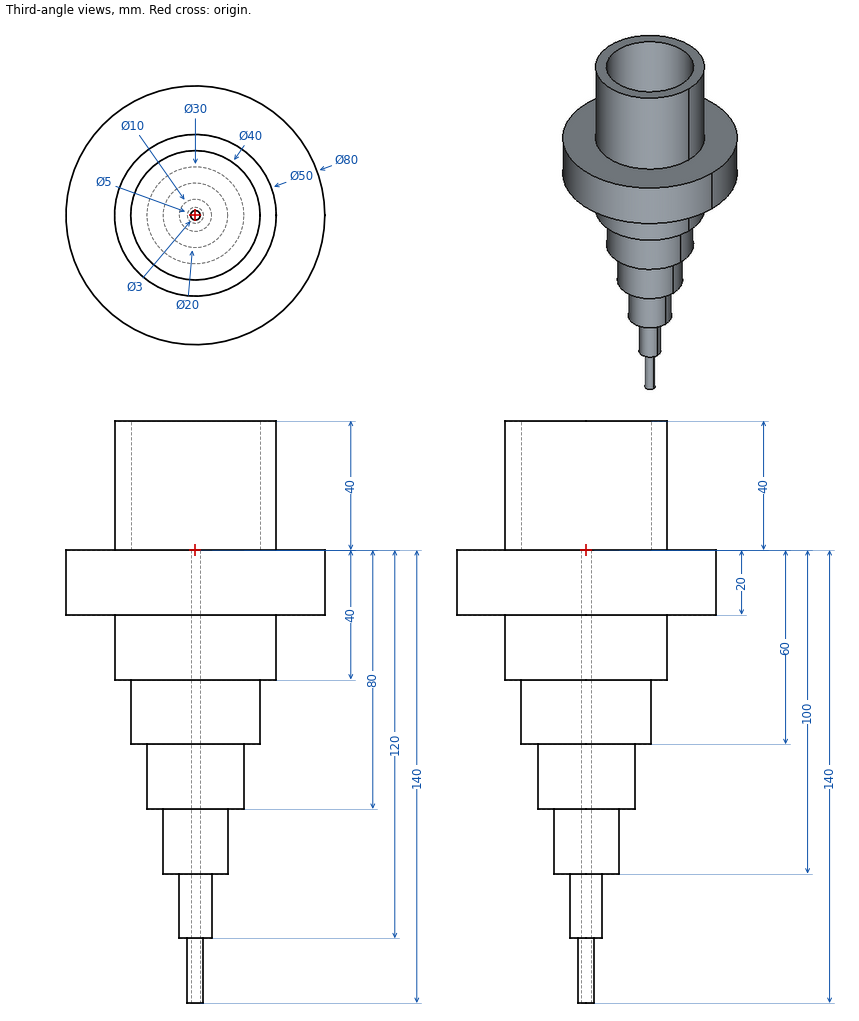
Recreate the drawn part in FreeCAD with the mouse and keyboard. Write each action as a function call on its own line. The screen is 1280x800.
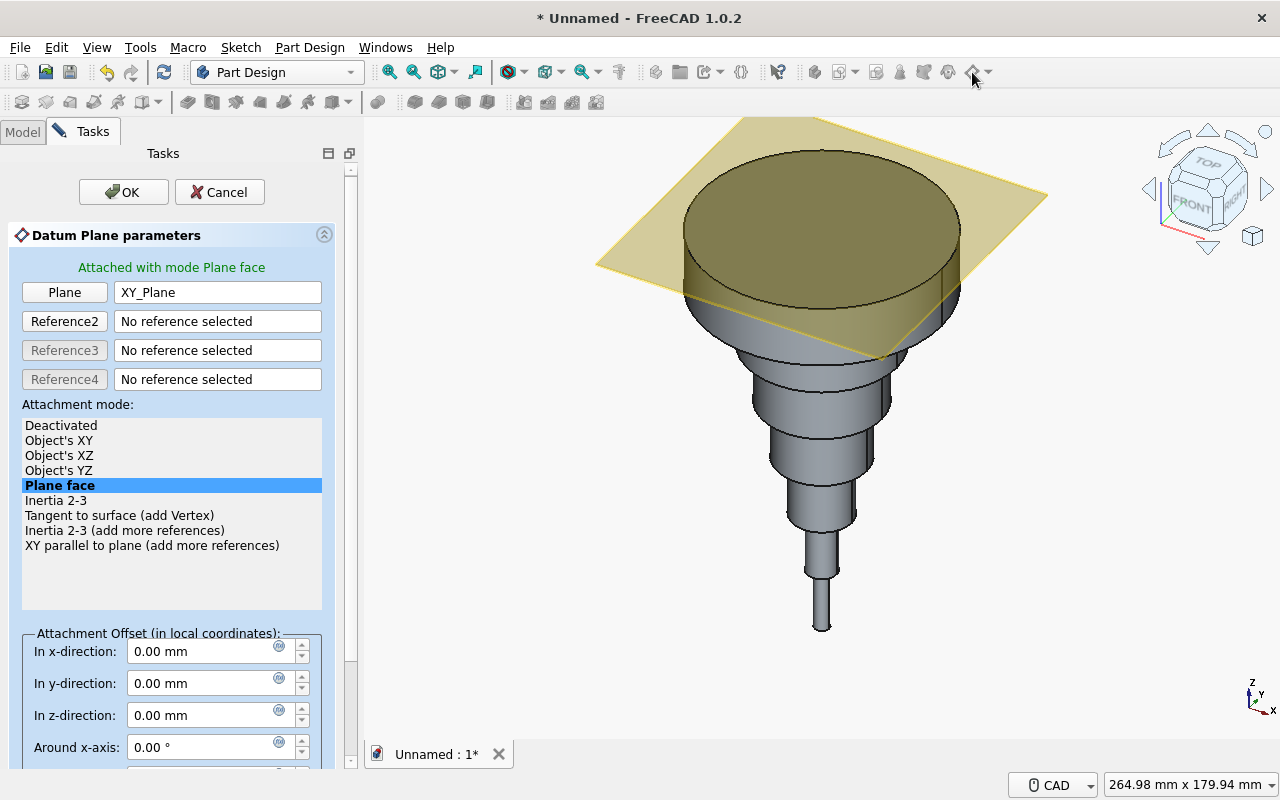
triple_click(210, 715)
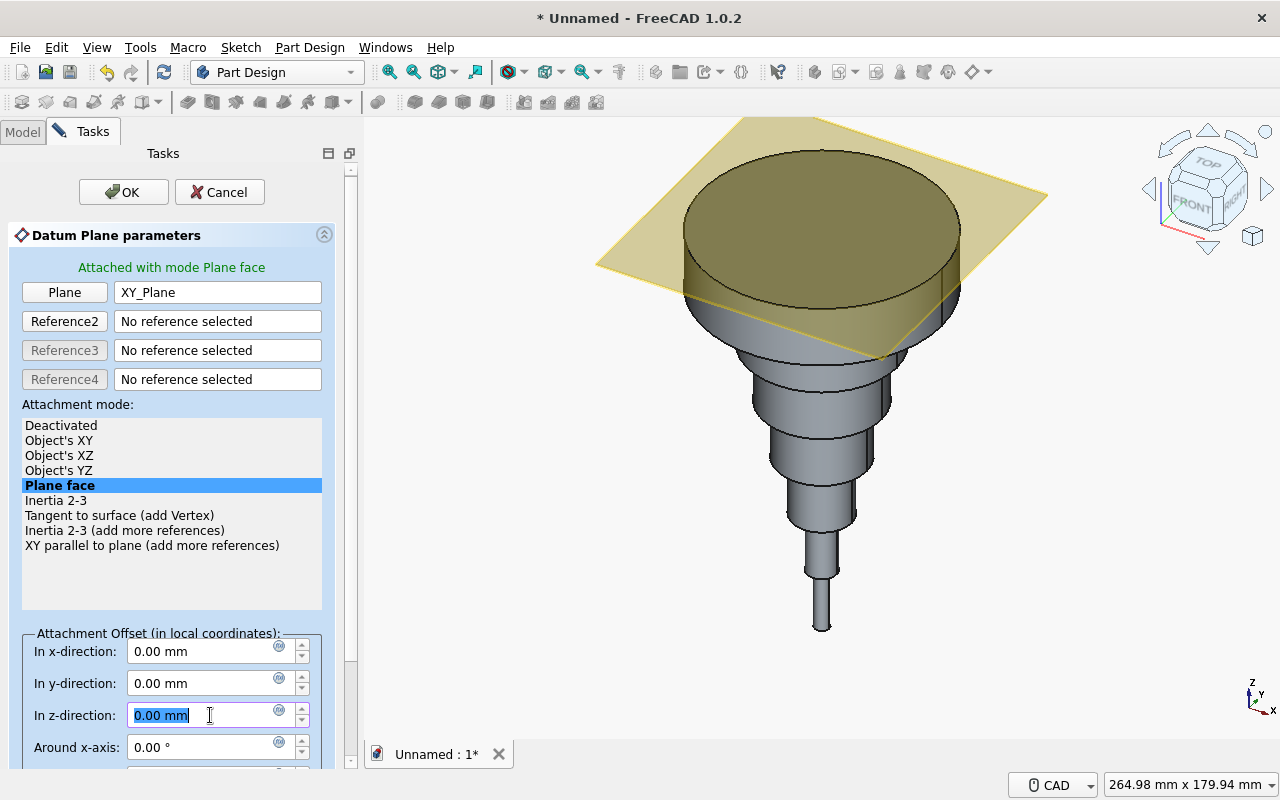
text(40)
key(Tab)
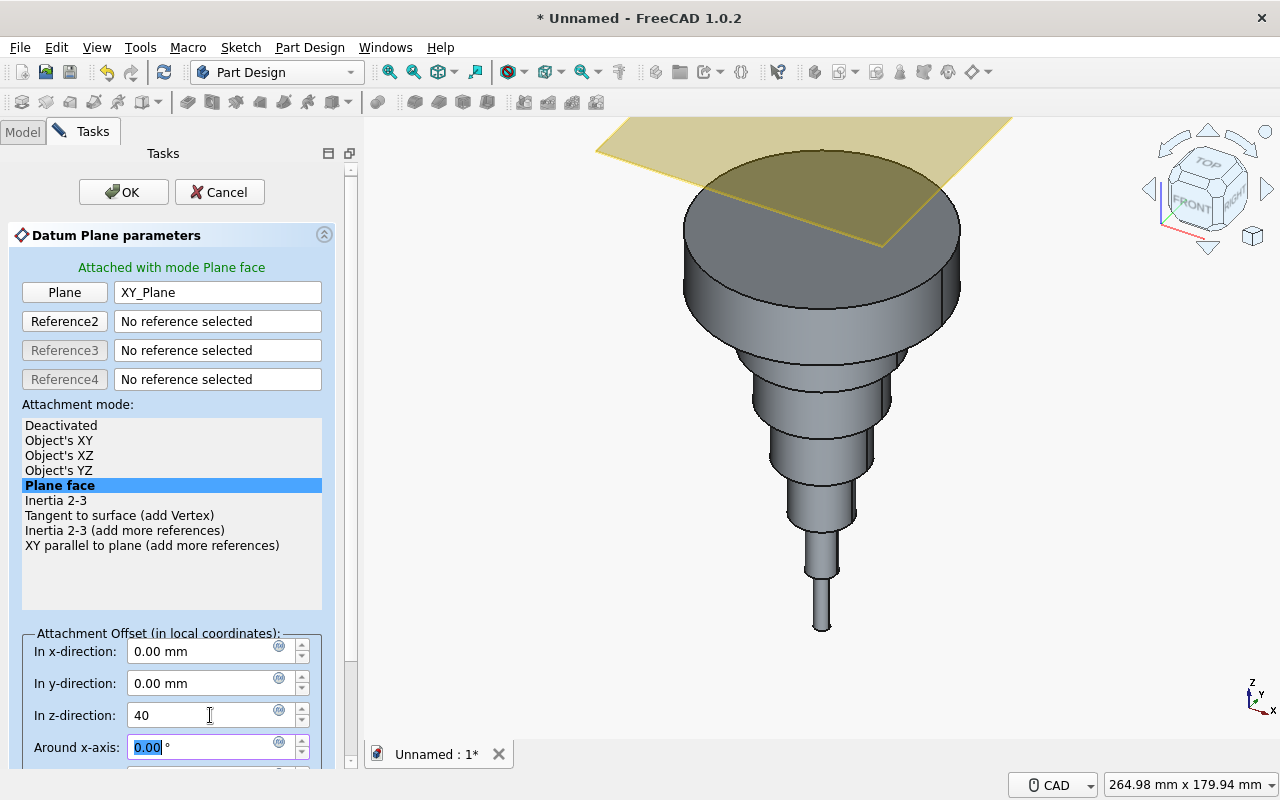
click(124, 192)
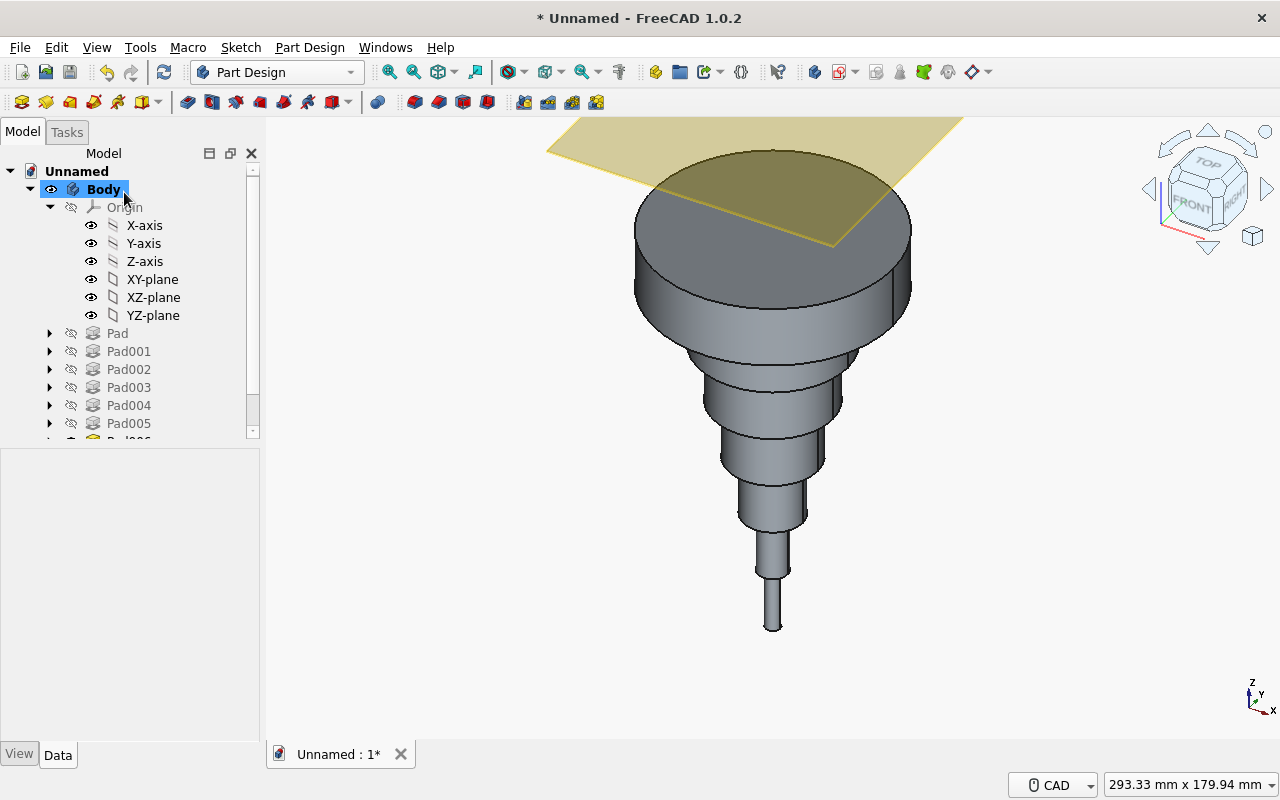
scroll(100, 293, down, 3)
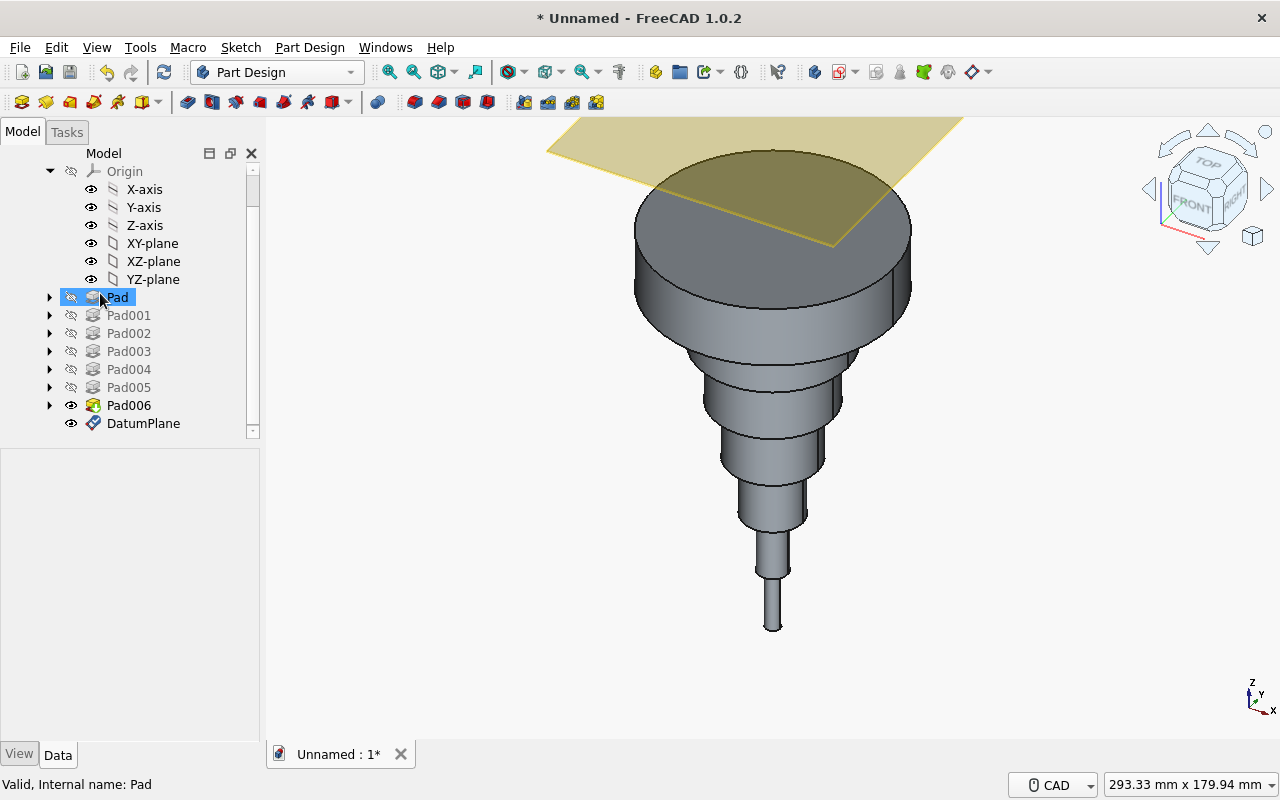
click(116, 423)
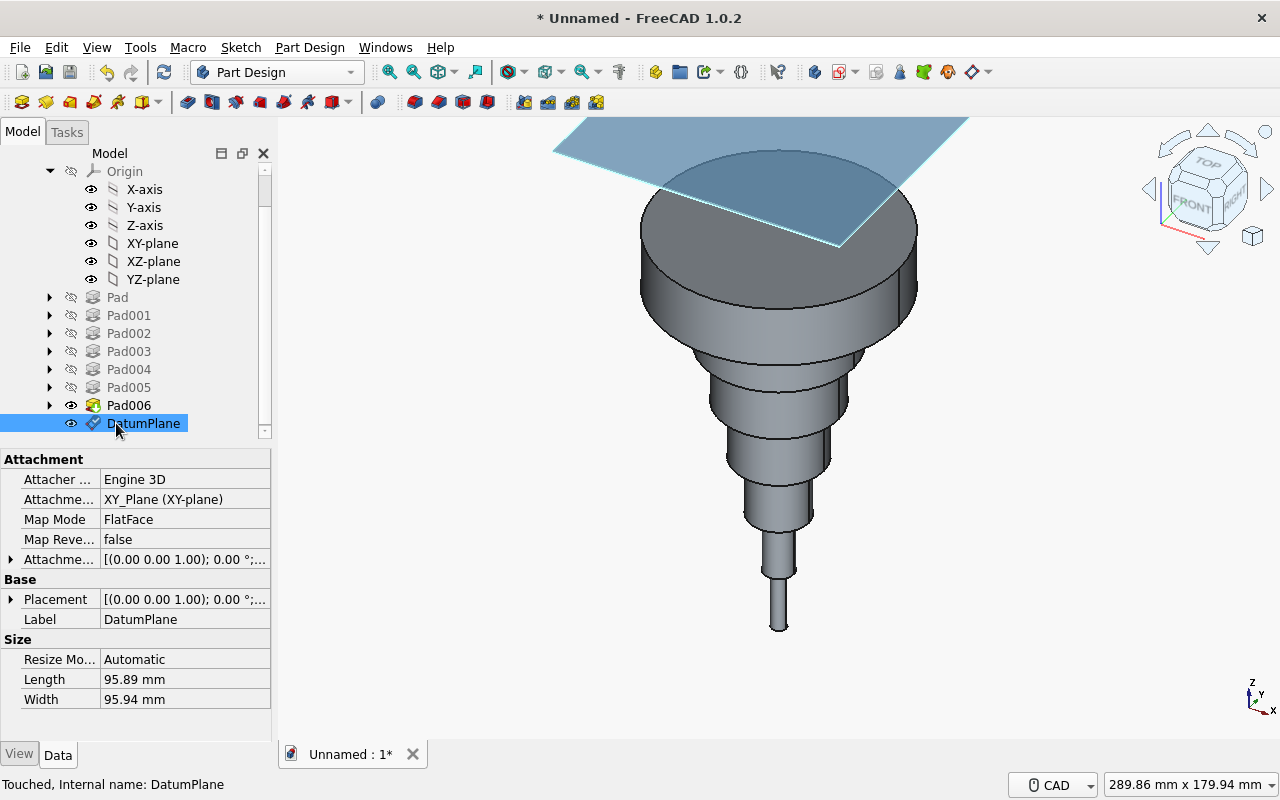
click(840, 72)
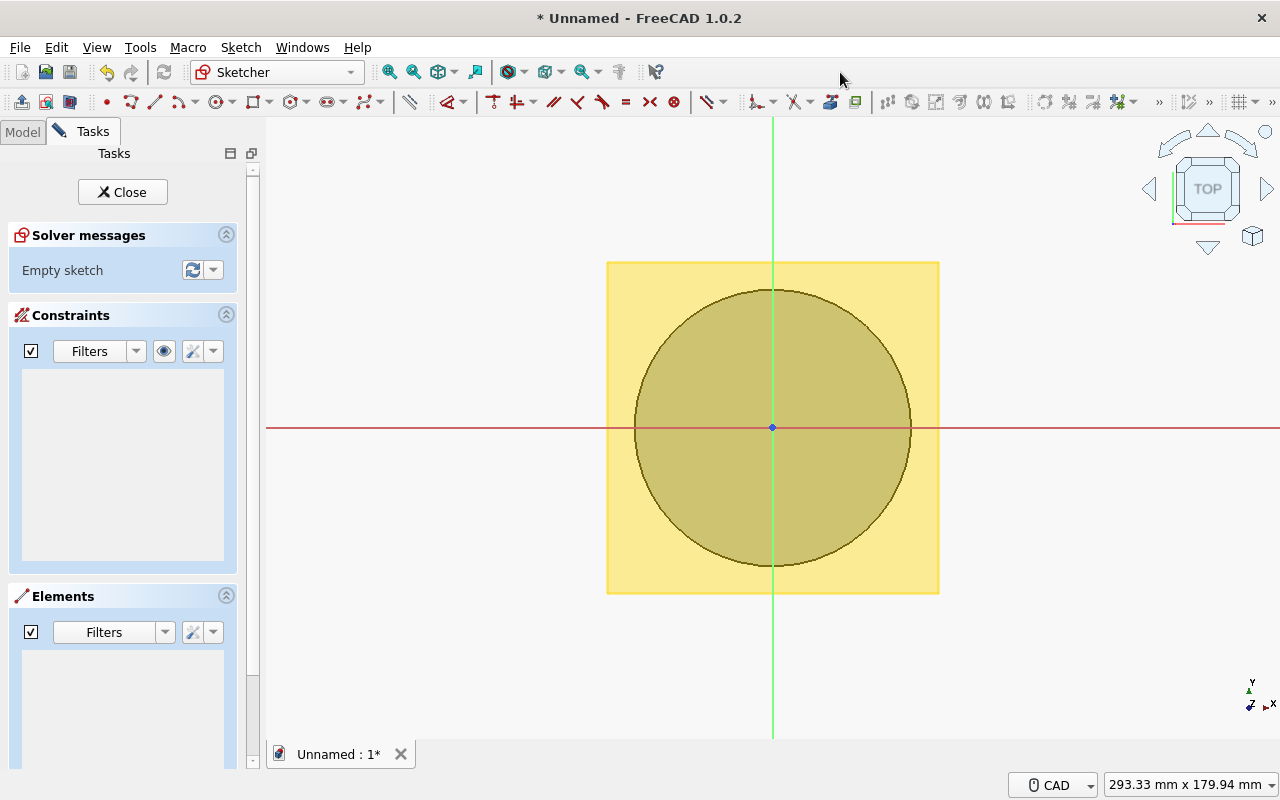
scroll(829, 428, up, 4)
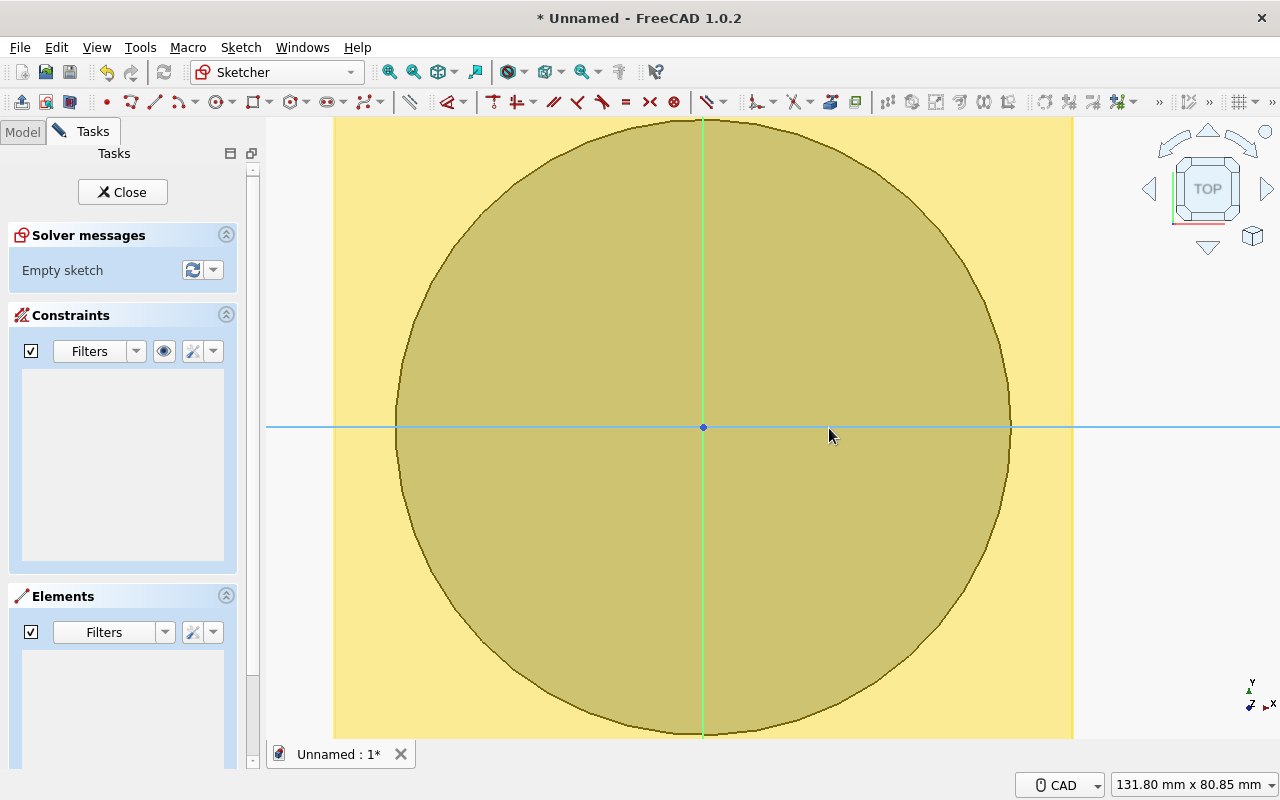
click(216, 102)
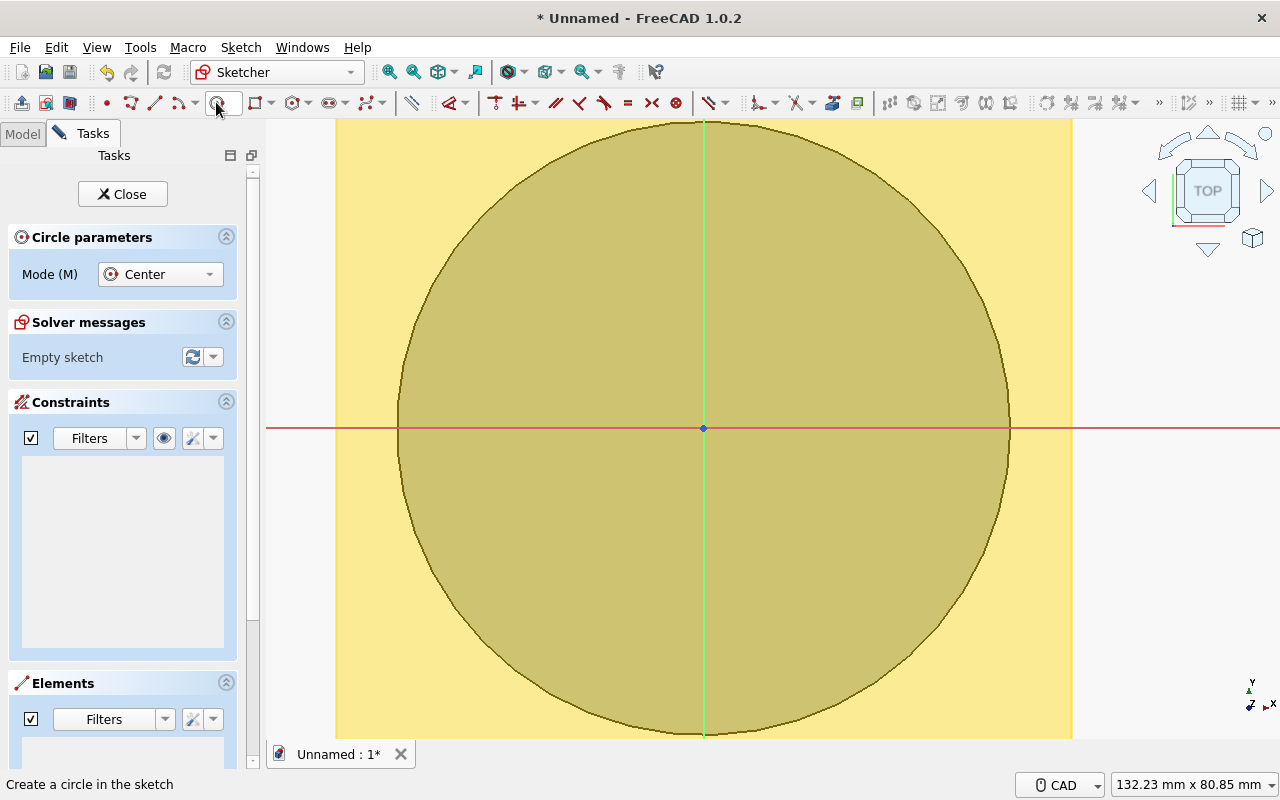
click(704, 428)
move(839, 293)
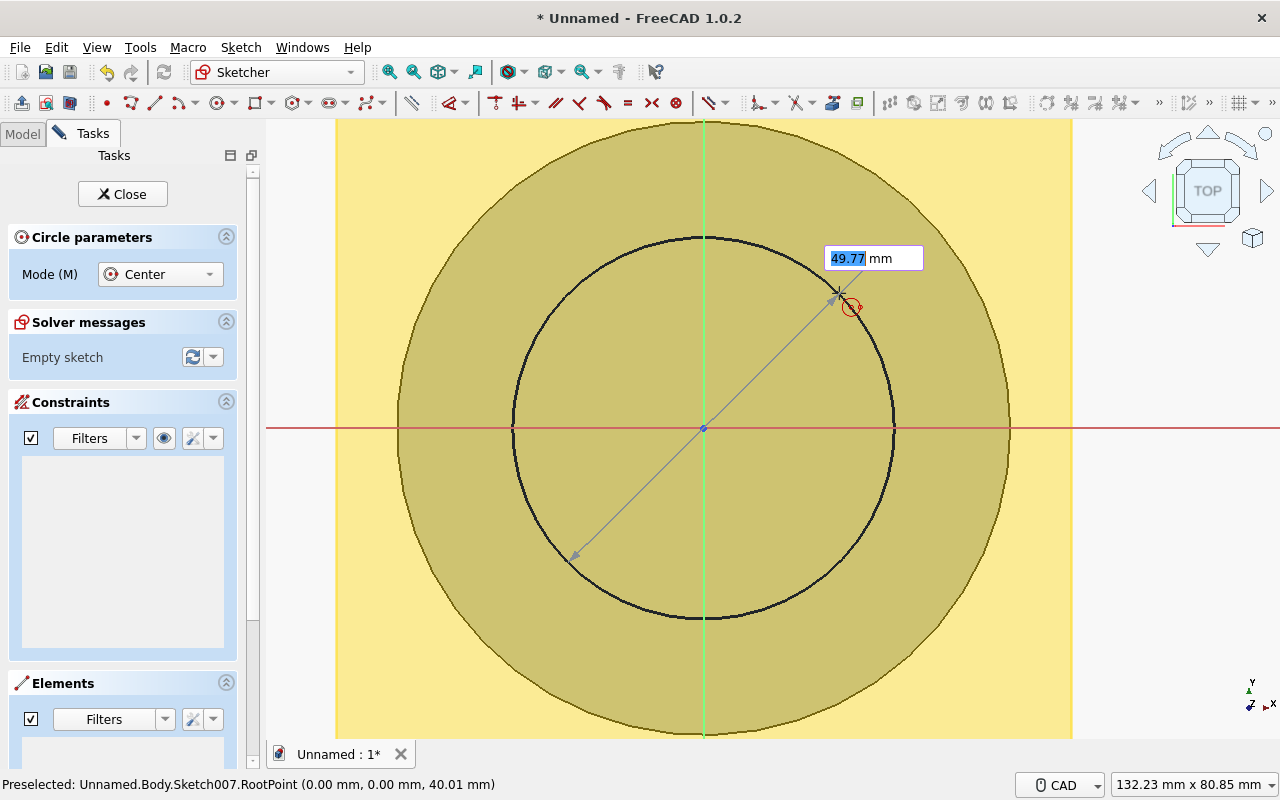
text(50)
key(Return)
key(Escape)